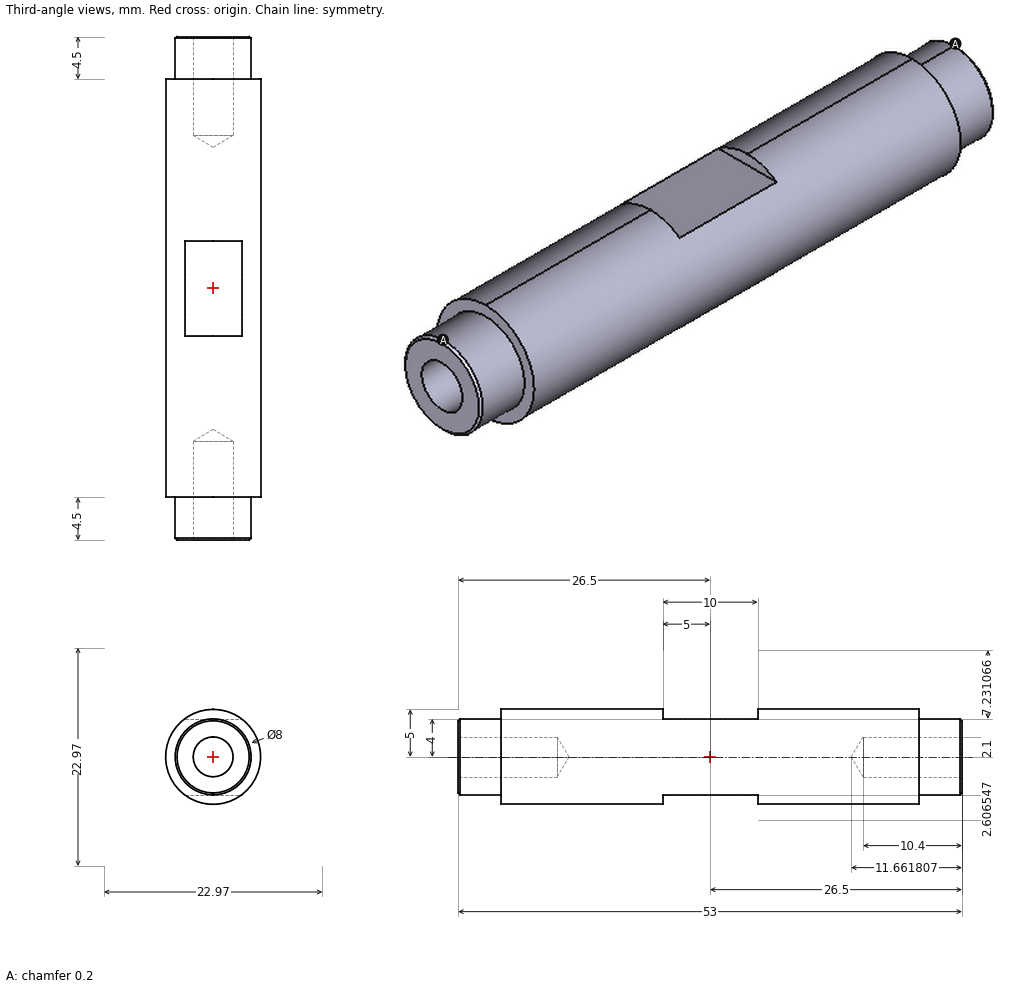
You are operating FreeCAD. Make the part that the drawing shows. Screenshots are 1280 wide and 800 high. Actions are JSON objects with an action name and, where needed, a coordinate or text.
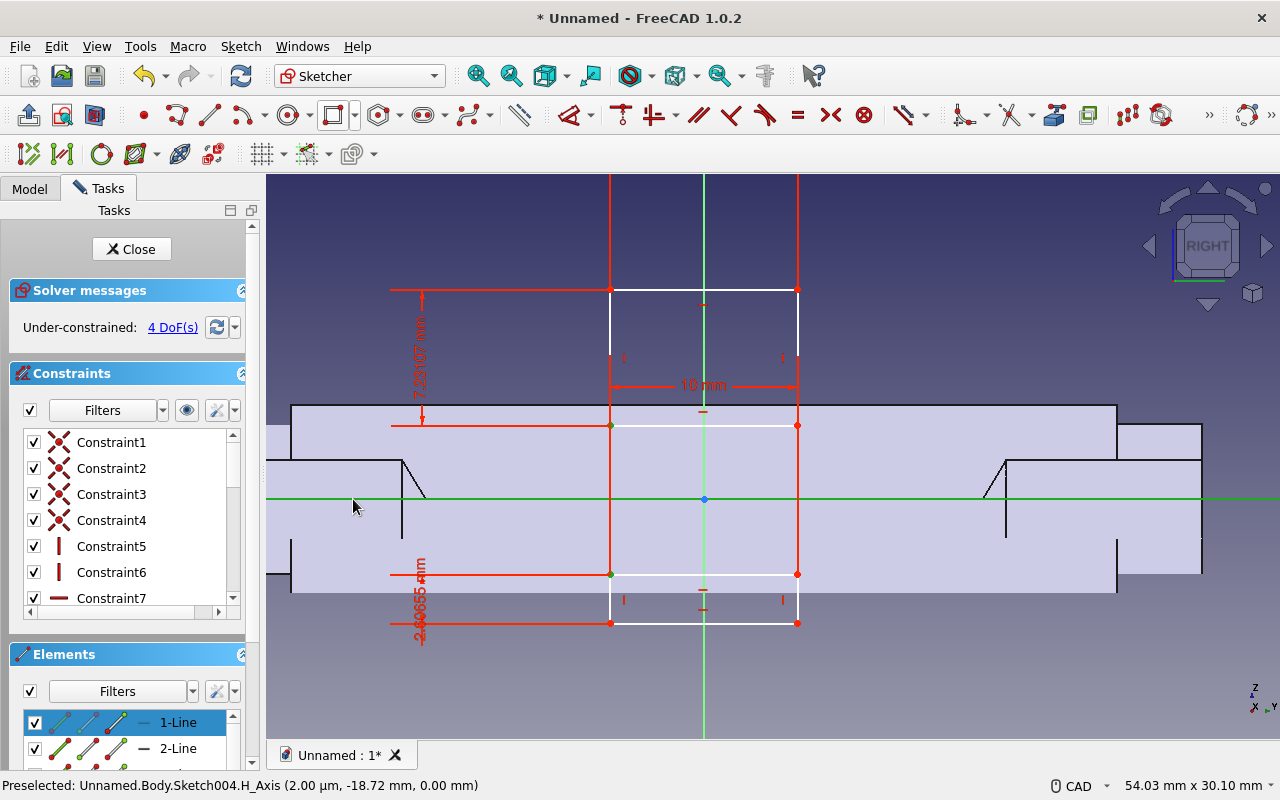
{"action": "left_click", "coordinate": [831, 116]}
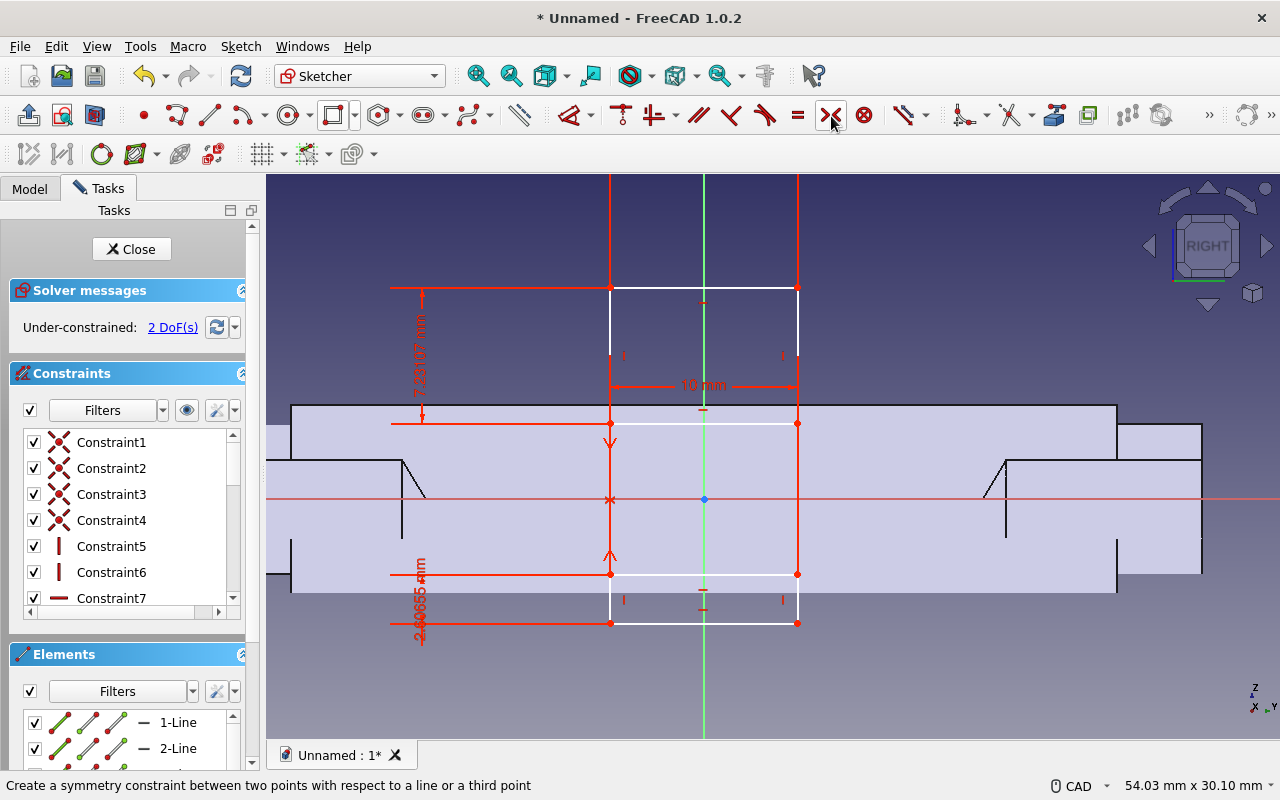
{"action": "left_click", "coordinate": [568, 116]}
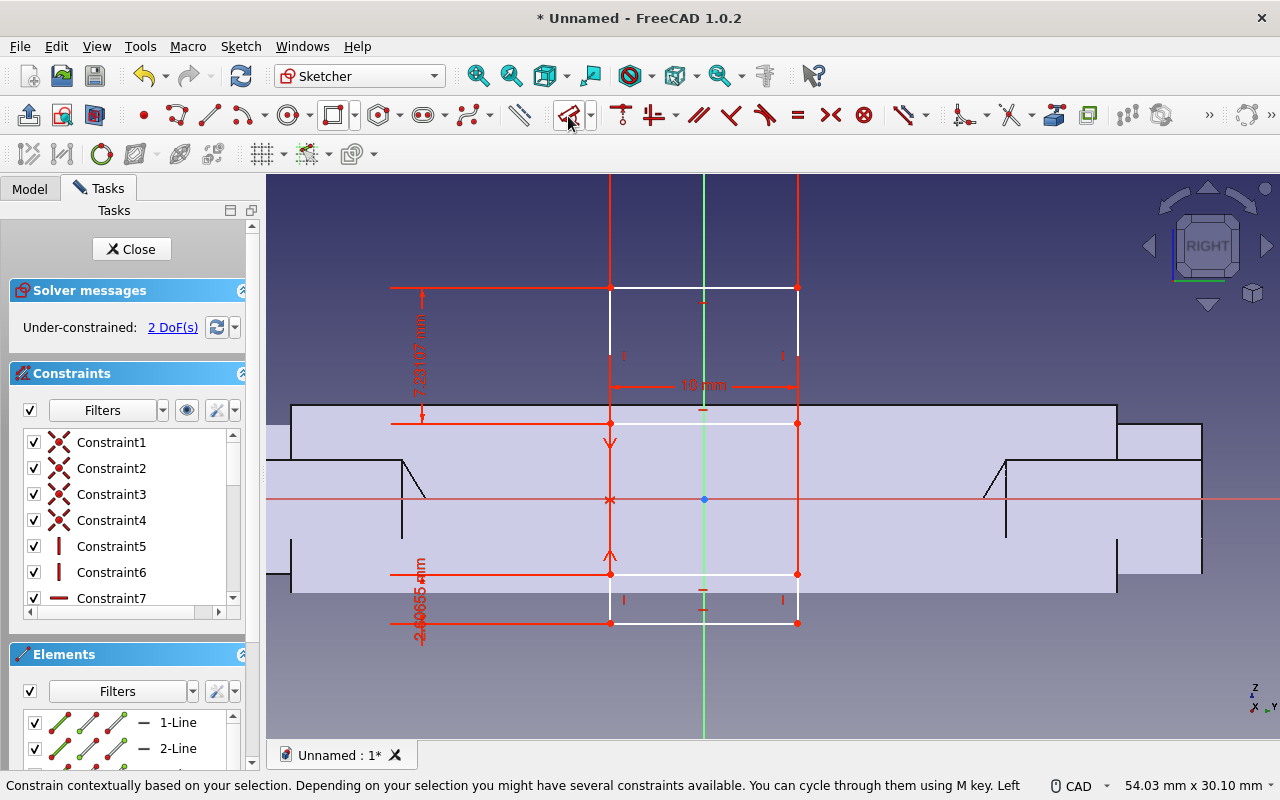
{"action": "left_click", "coordinate": [610, 288]}
{"action": "left_click", "coordinate": [657, 254]}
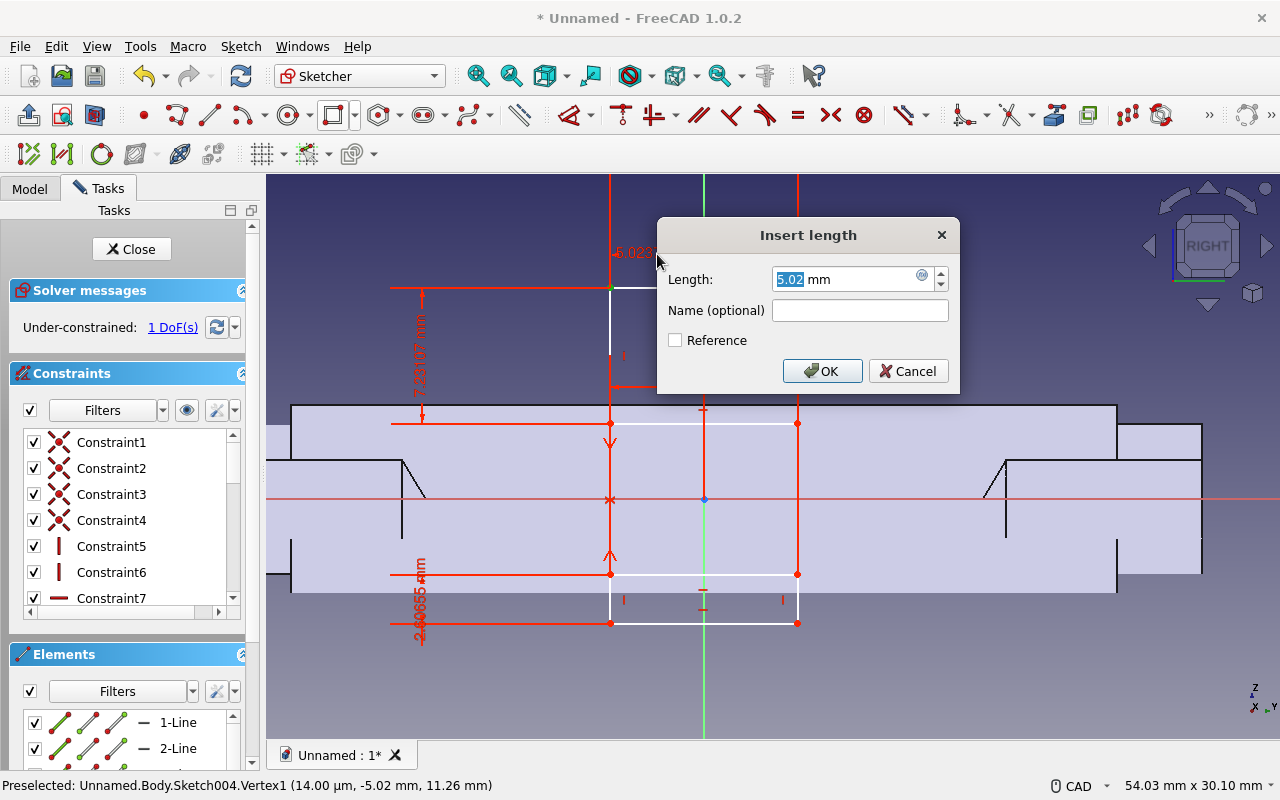
{"action": "type", "text": "5"}
{"action": "key", "text": "Return"}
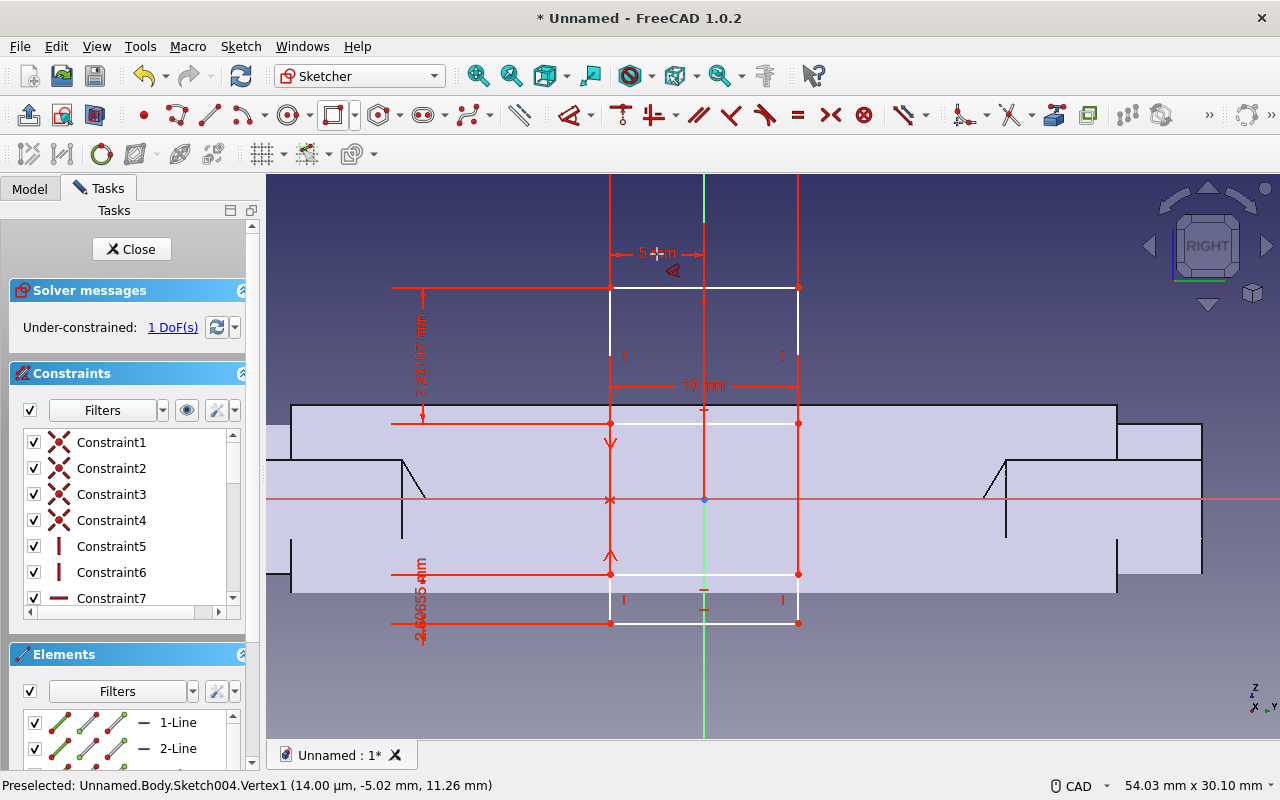
{"action": "left_click", "coordinate": [610, 424]}
{"action": "left_click", "coordinate": [576, 461]}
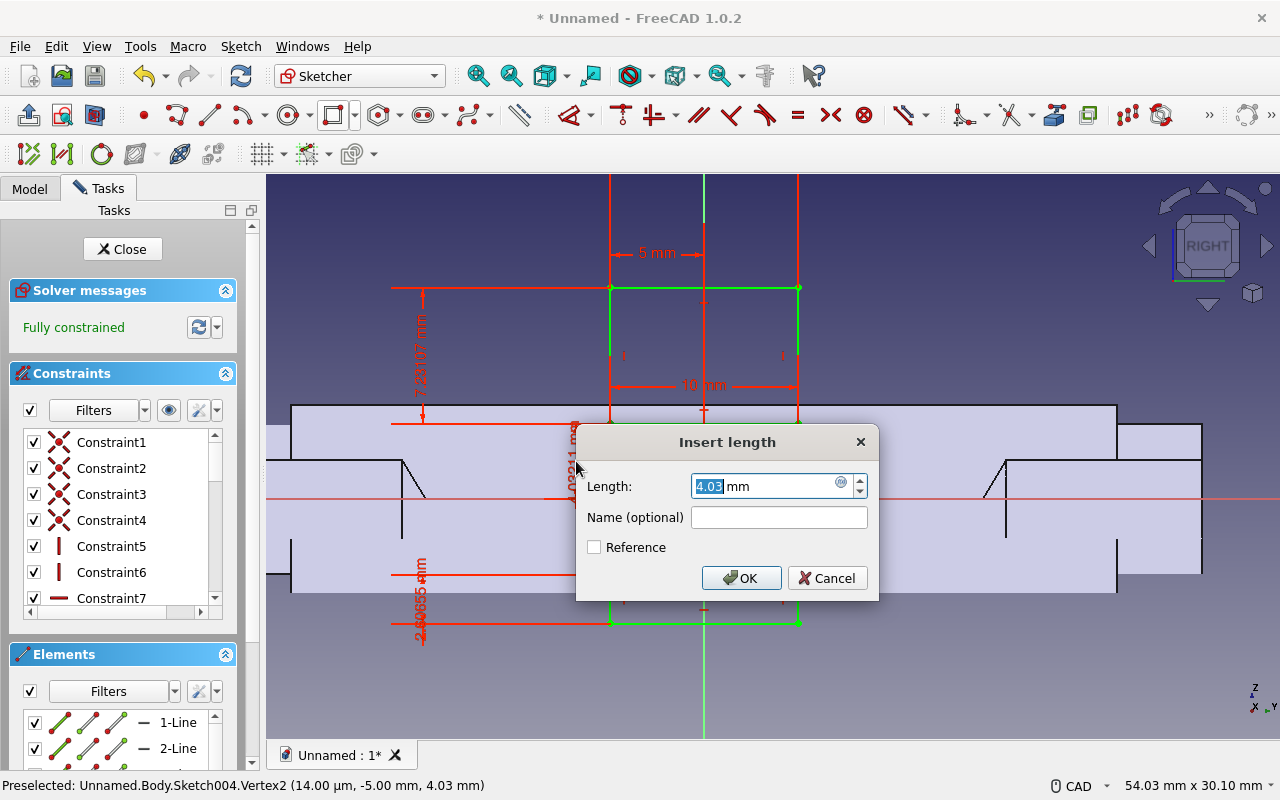
{"action": "type", "text": "4"}
{"action": "key", "text": "Return"}
{"action": "key", "text": "Escape"}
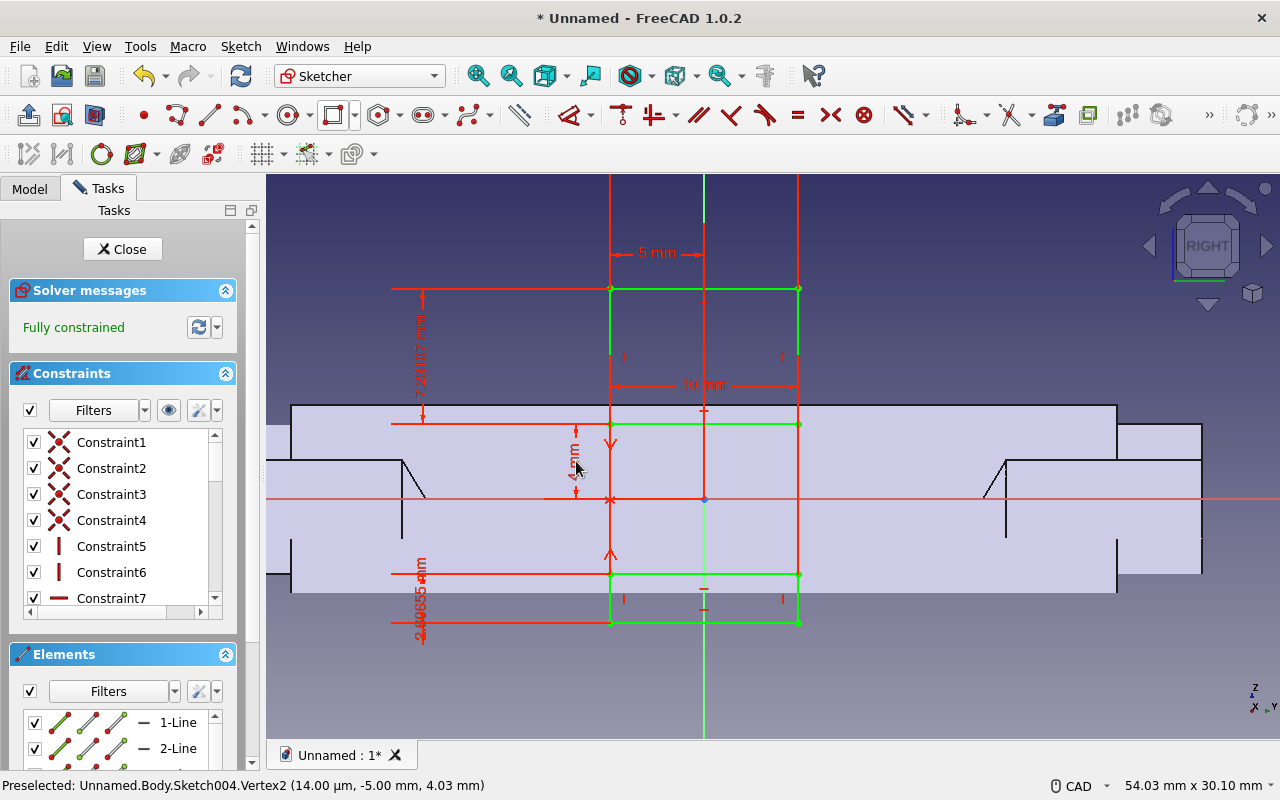
{"action": "left_click", "coordinate": [123, 249]}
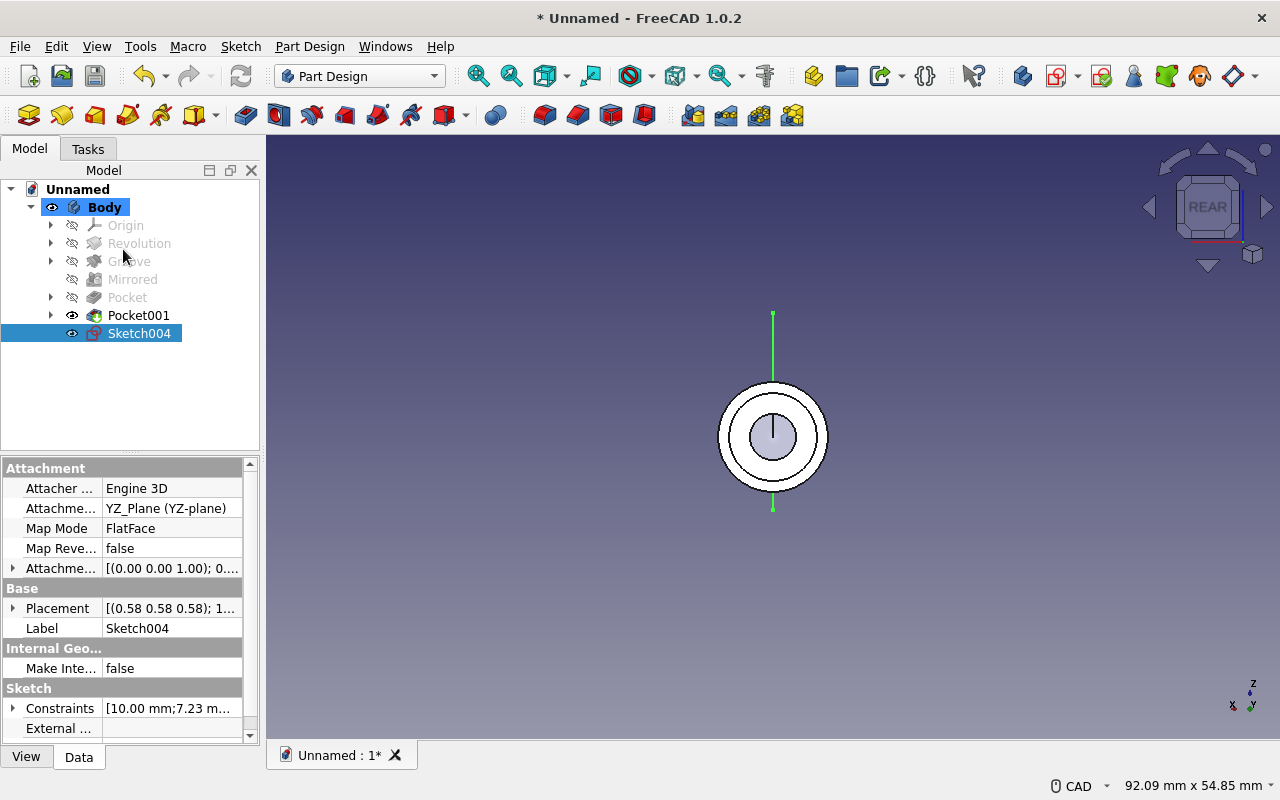
{"action": "left_click", "coordinate": [246, 116]}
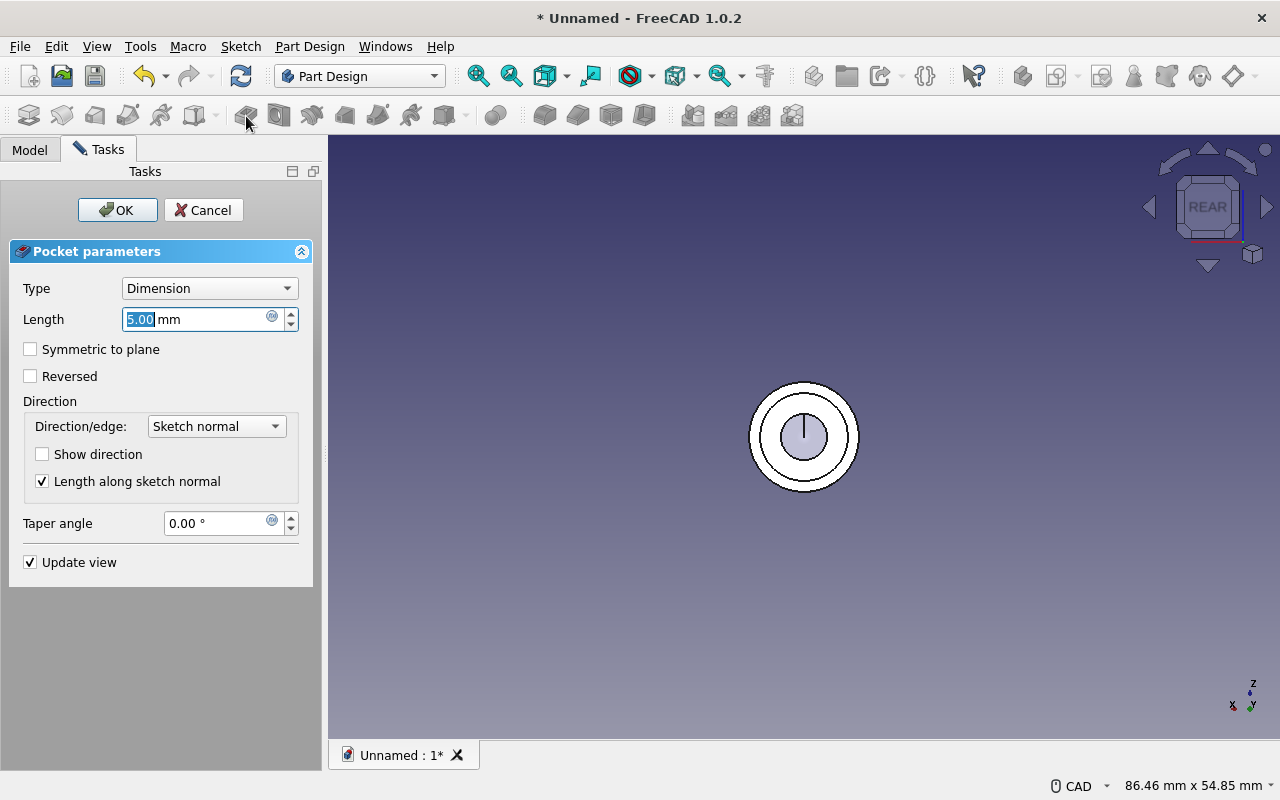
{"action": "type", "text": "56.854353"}
{"action": "key", "text": "Tab"}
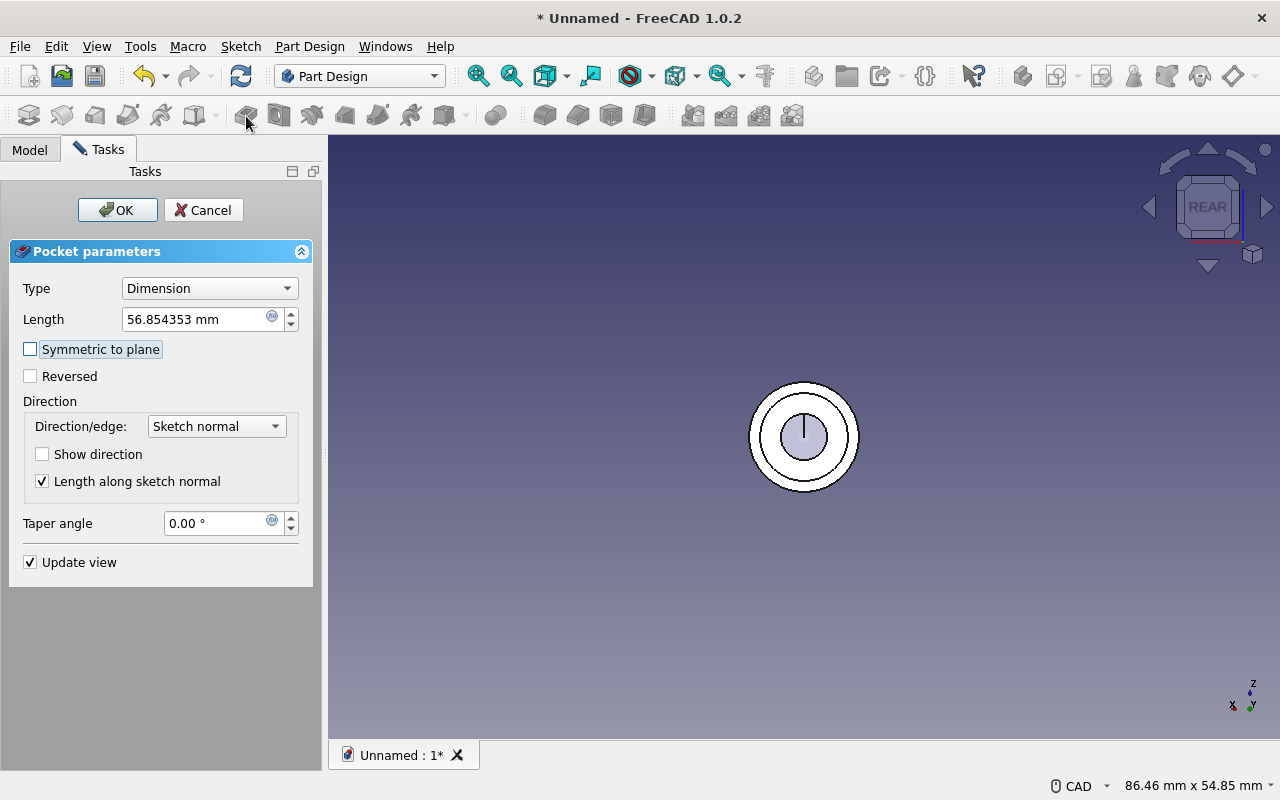
{"action": "left_click", "coordinate": [31, 349]}